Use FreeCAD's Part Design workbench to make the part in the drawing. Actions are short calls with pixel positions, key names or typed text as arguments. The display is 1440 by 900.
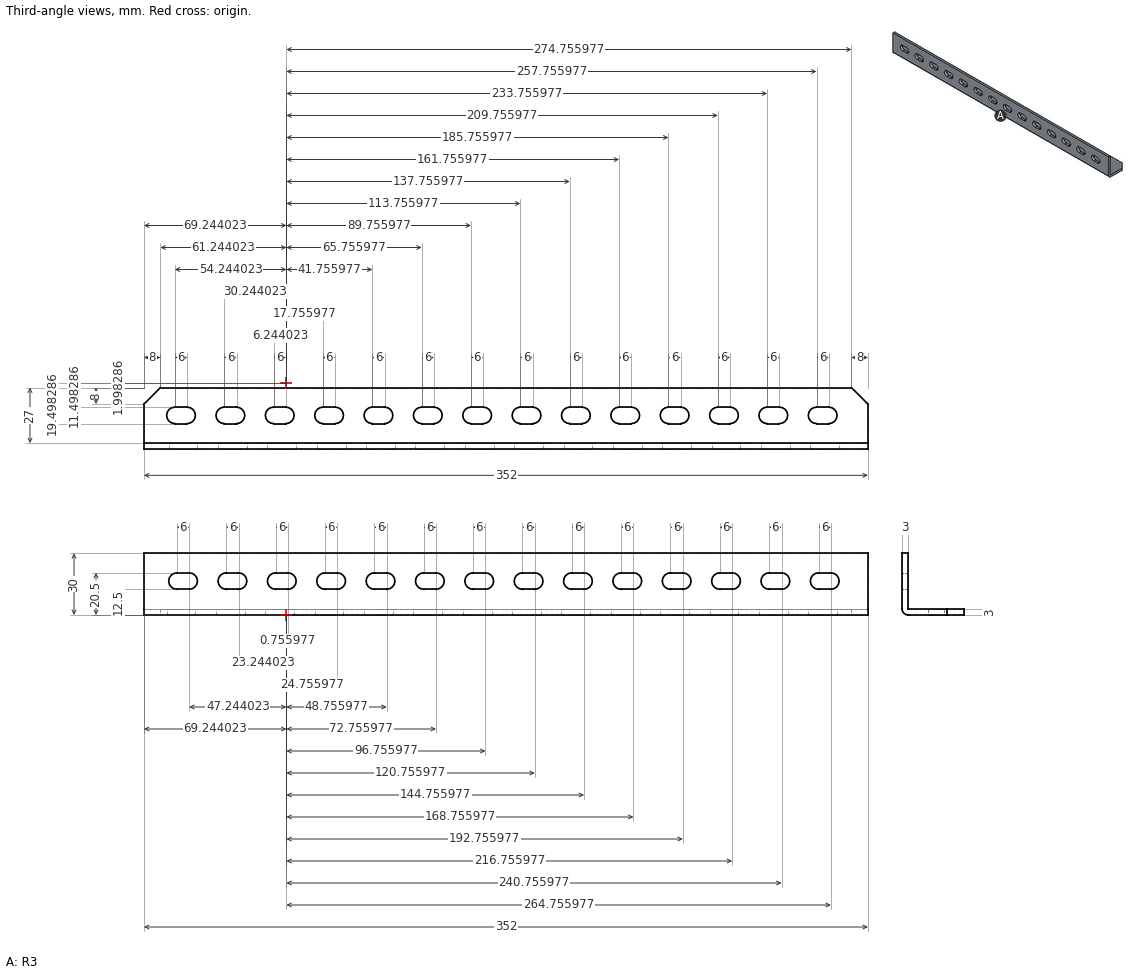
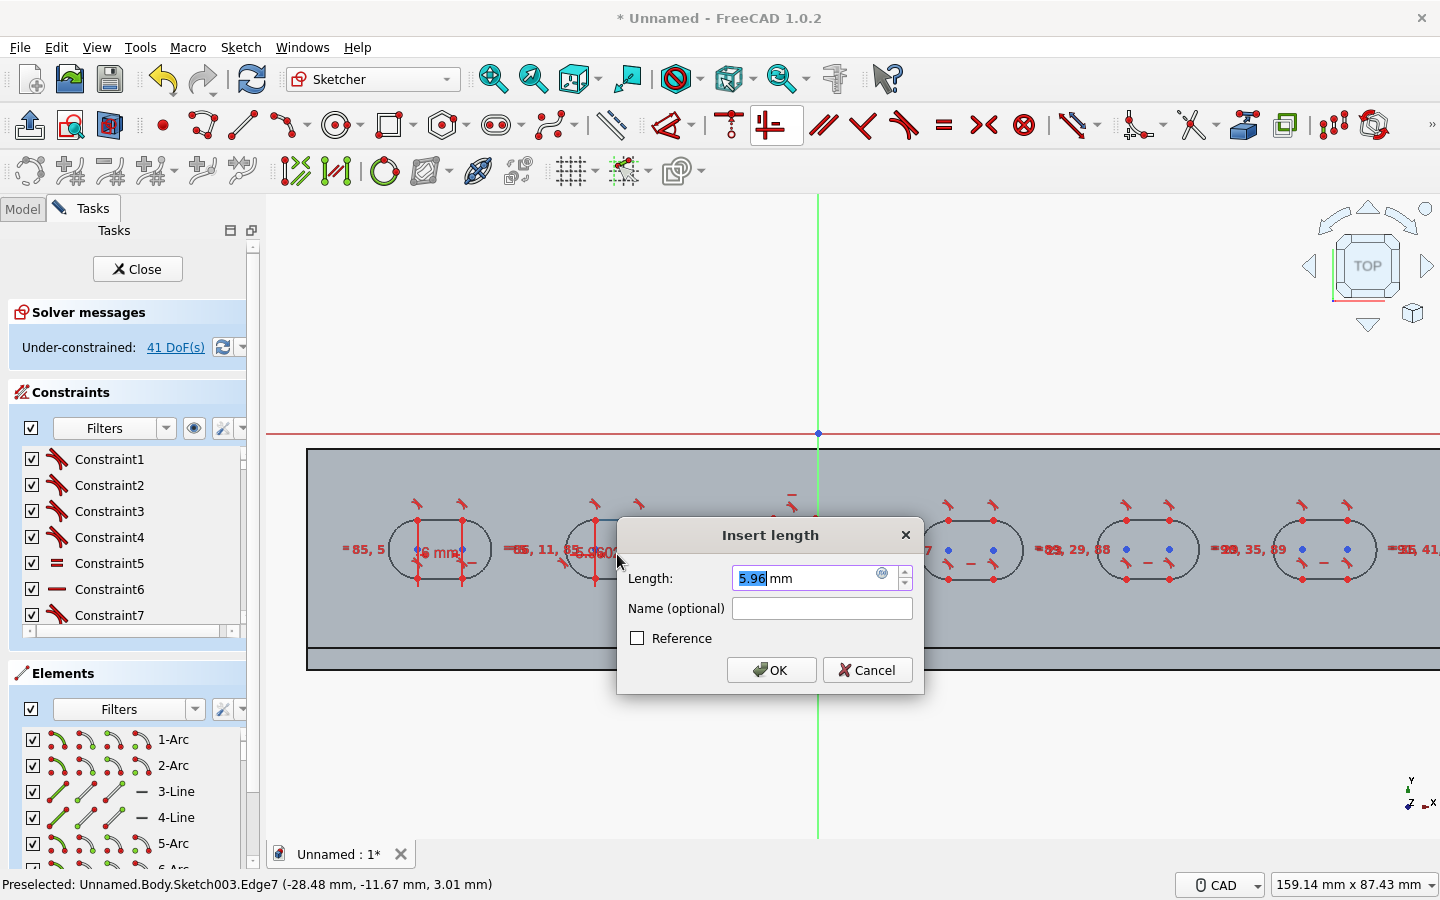
text(6)
key(Return)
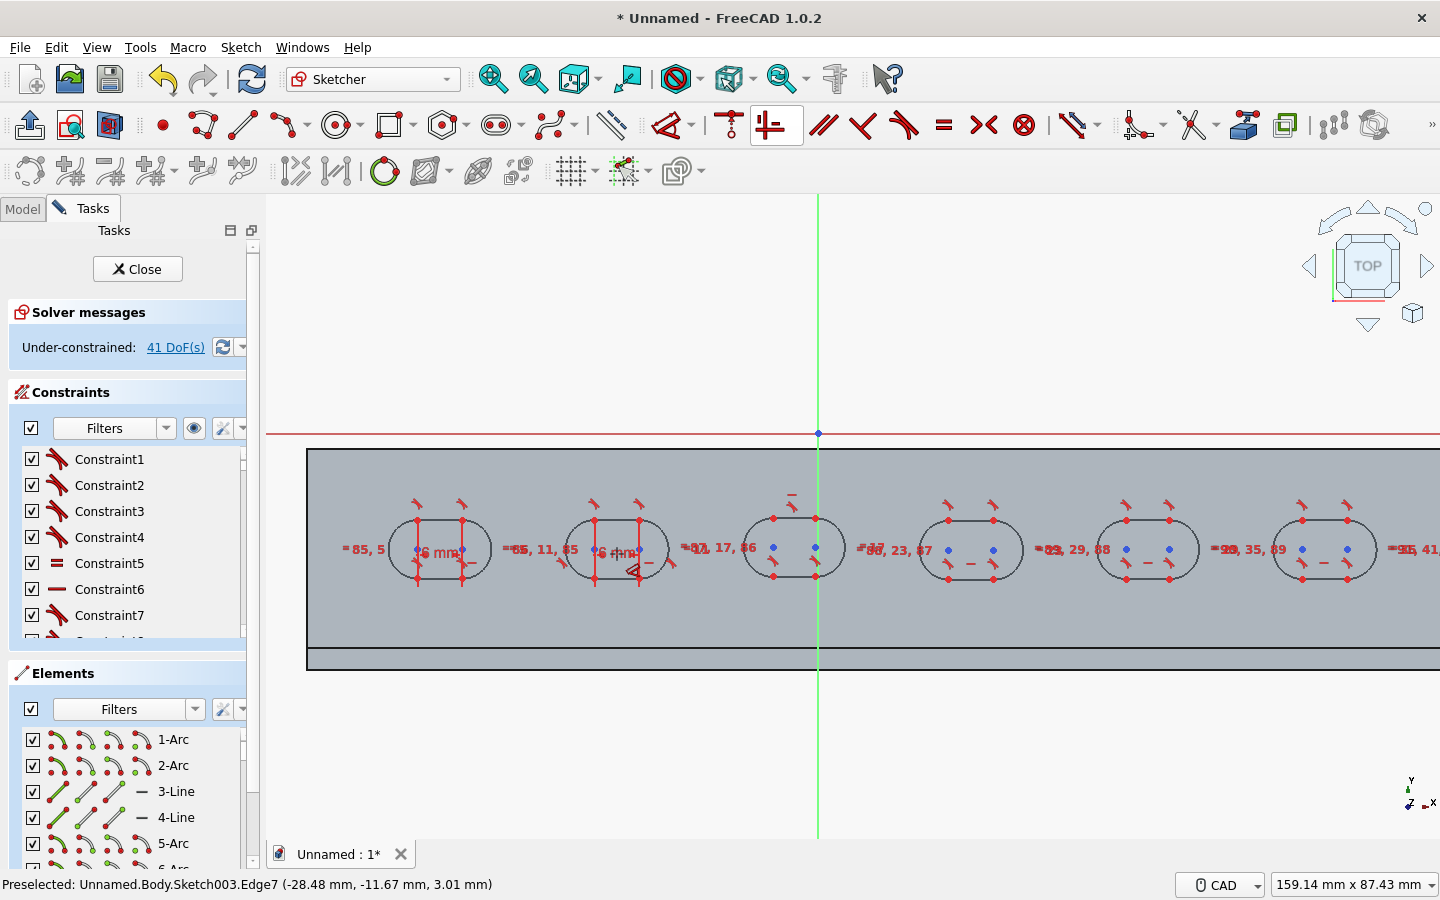
click(786, 518)
click(794, 552)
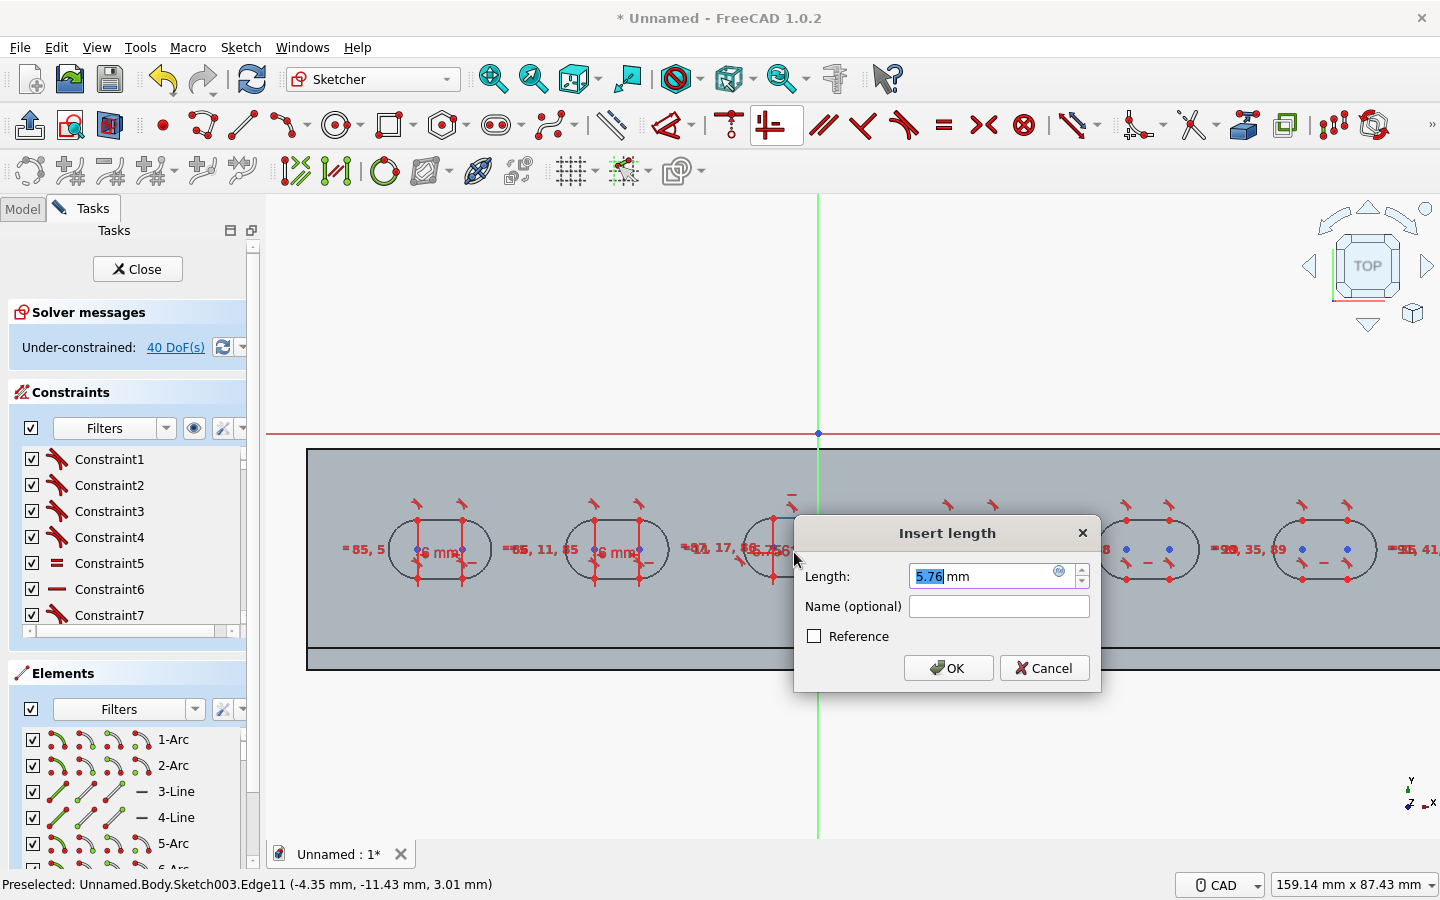
text(6)
key(Return)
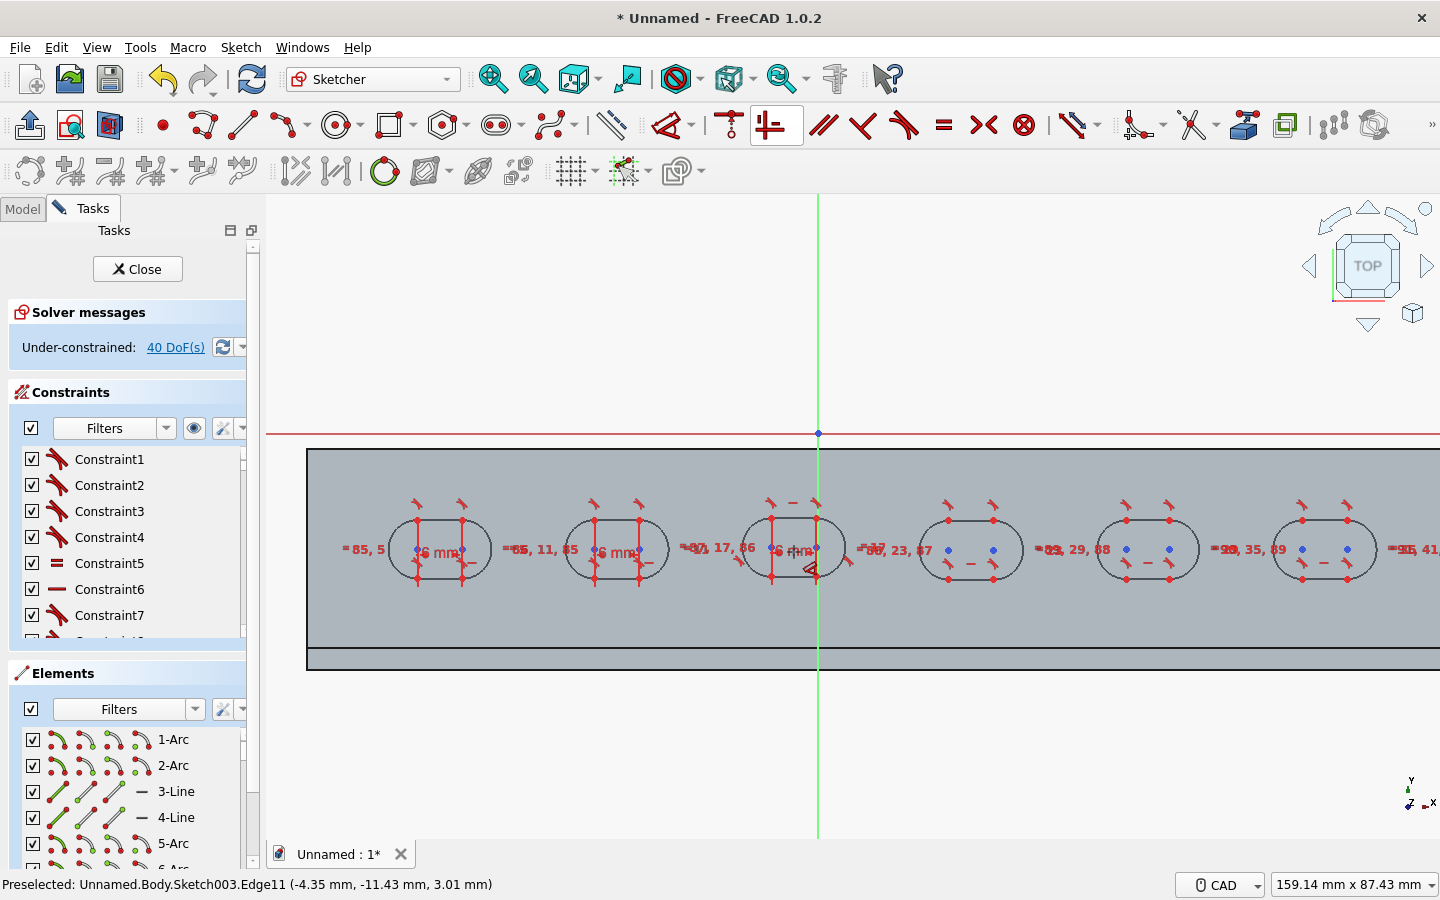
click(962, 521)
click(971, 555)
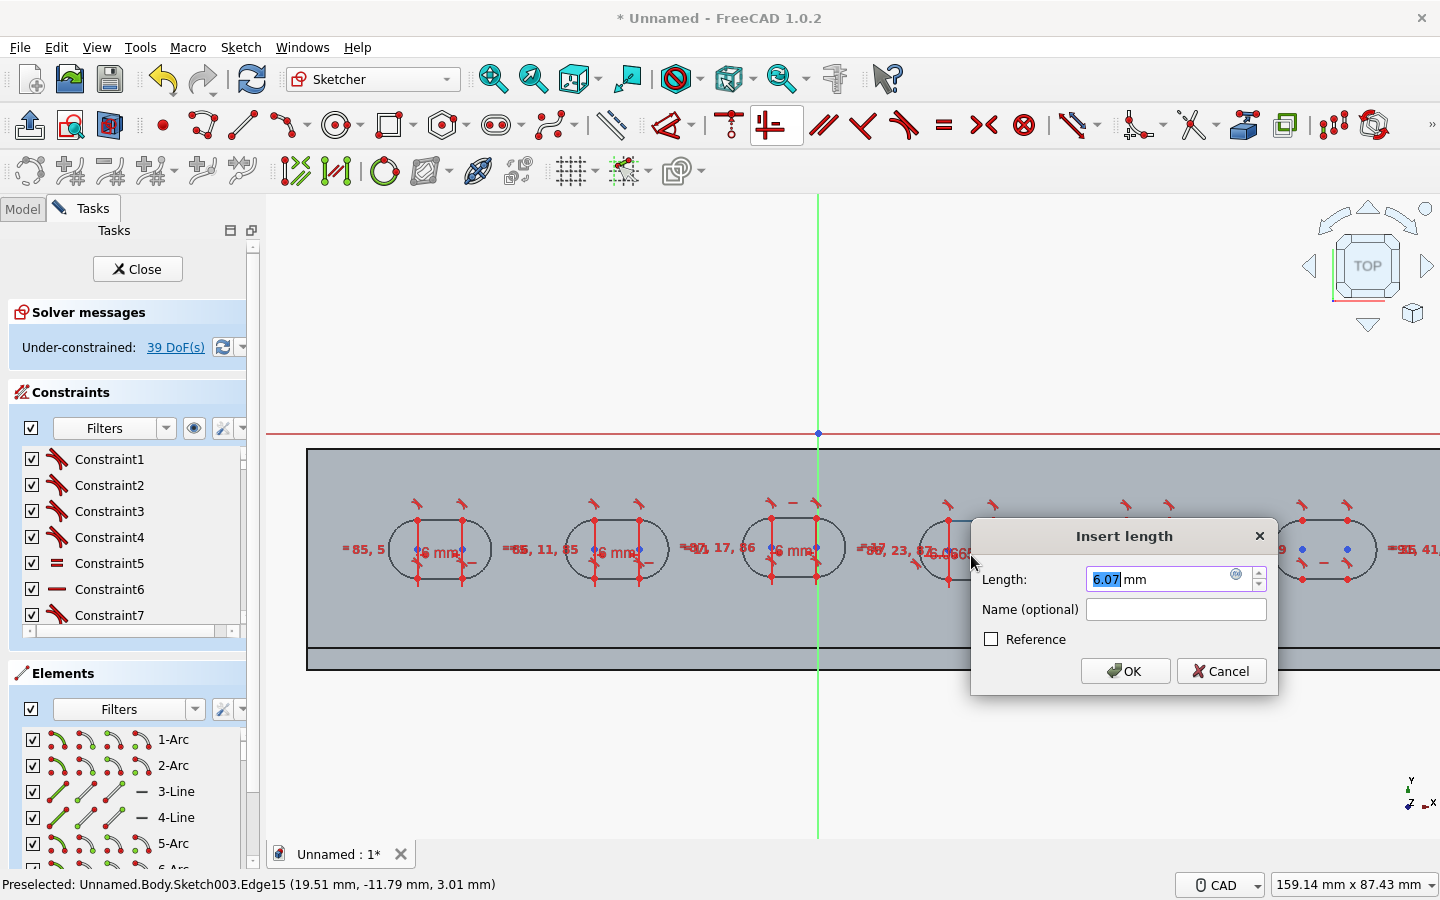
text(6)
key(Return)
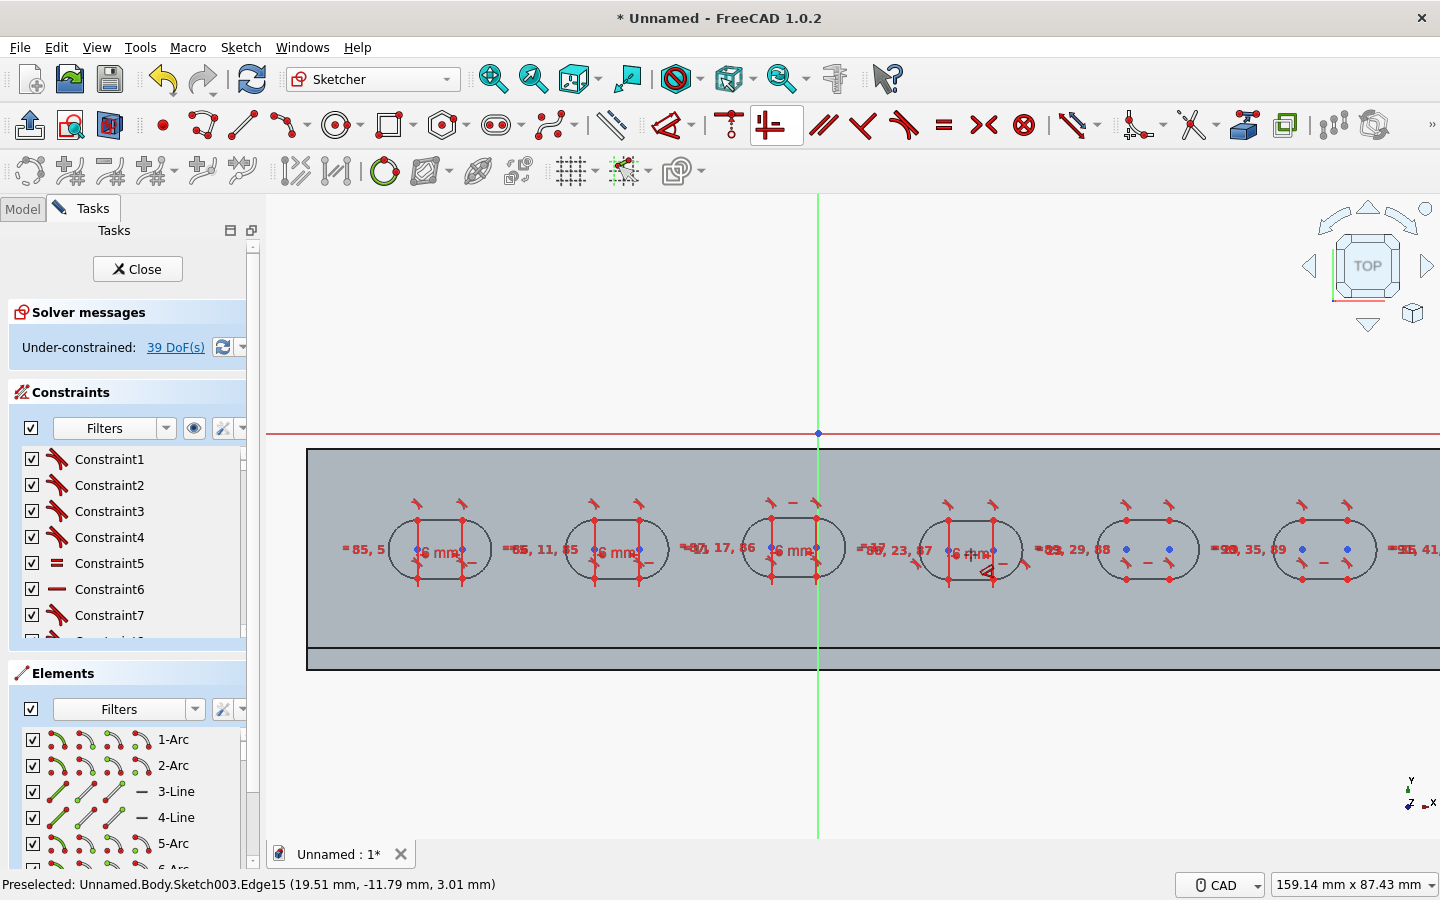
click(1139, 520)
click(1148, 554)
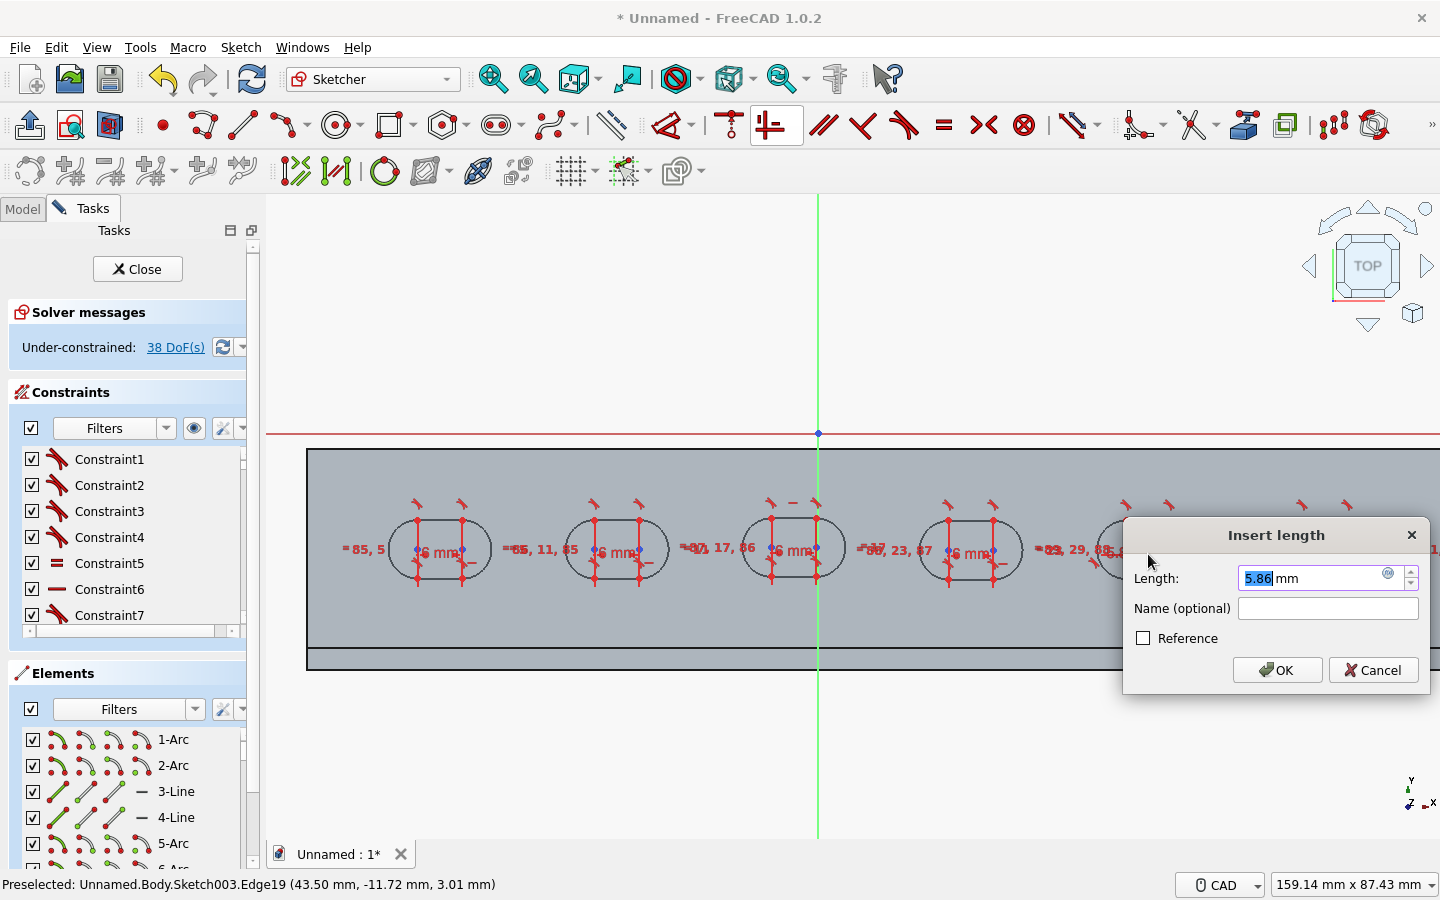
text(6)
key(Return)